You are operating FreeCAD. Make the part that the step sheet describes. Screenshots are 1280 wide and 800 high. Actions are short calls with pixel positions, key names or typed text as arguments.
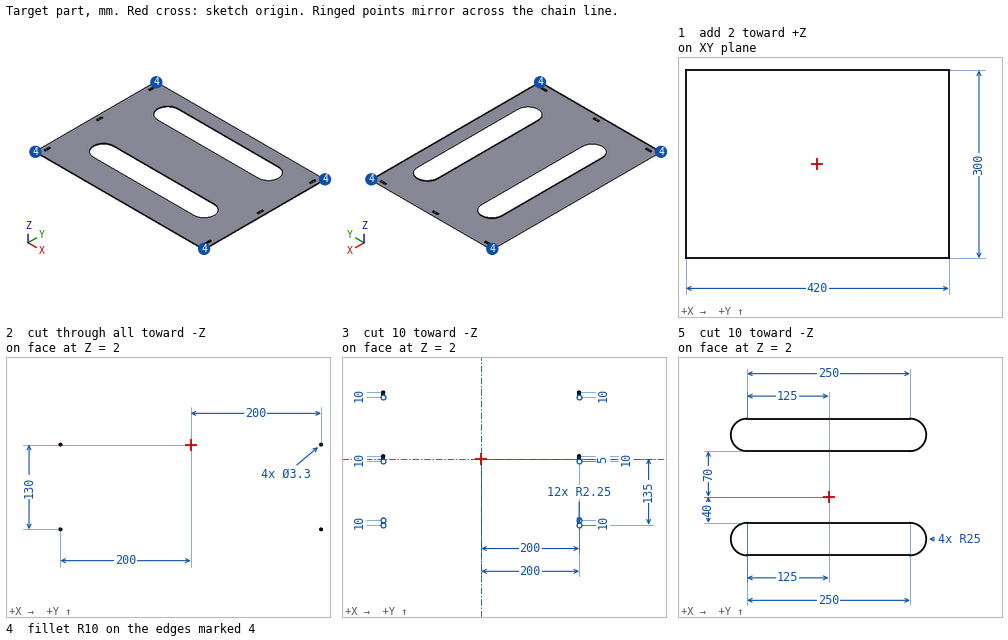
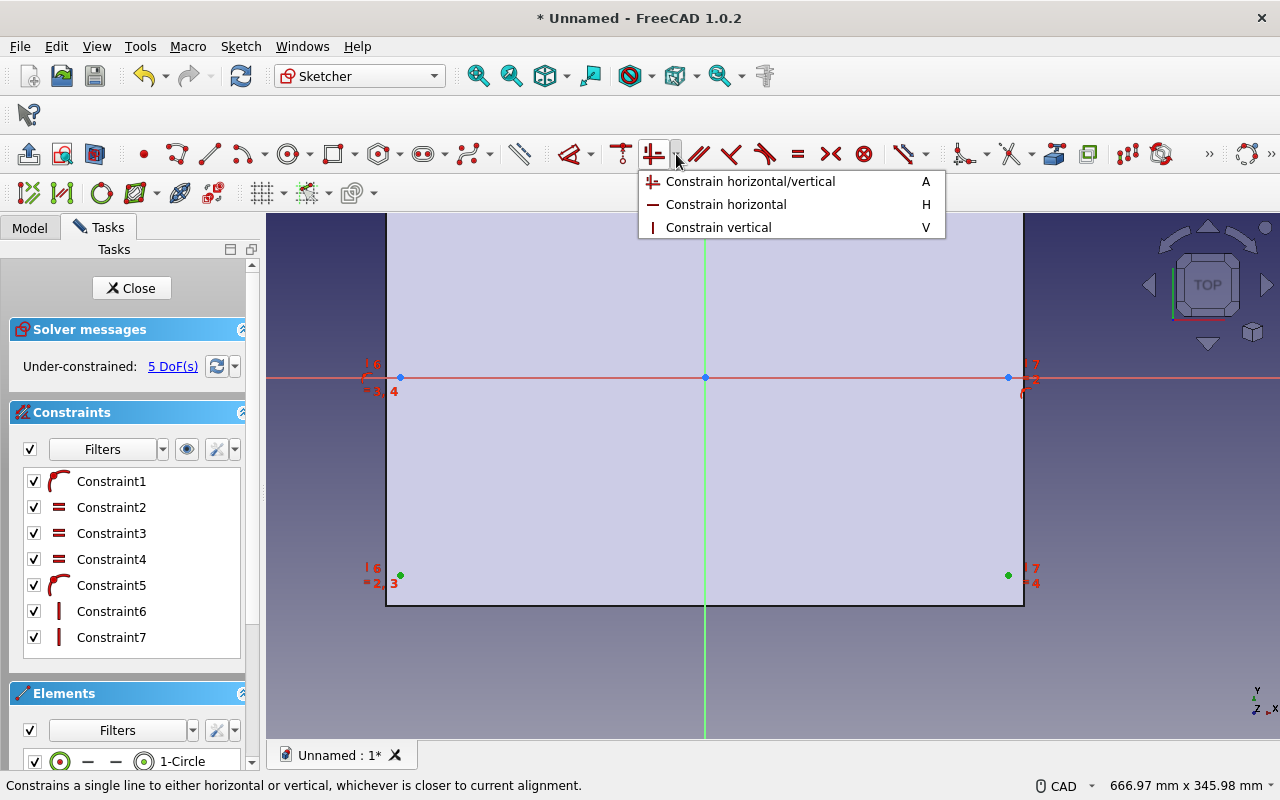
click(792, 204)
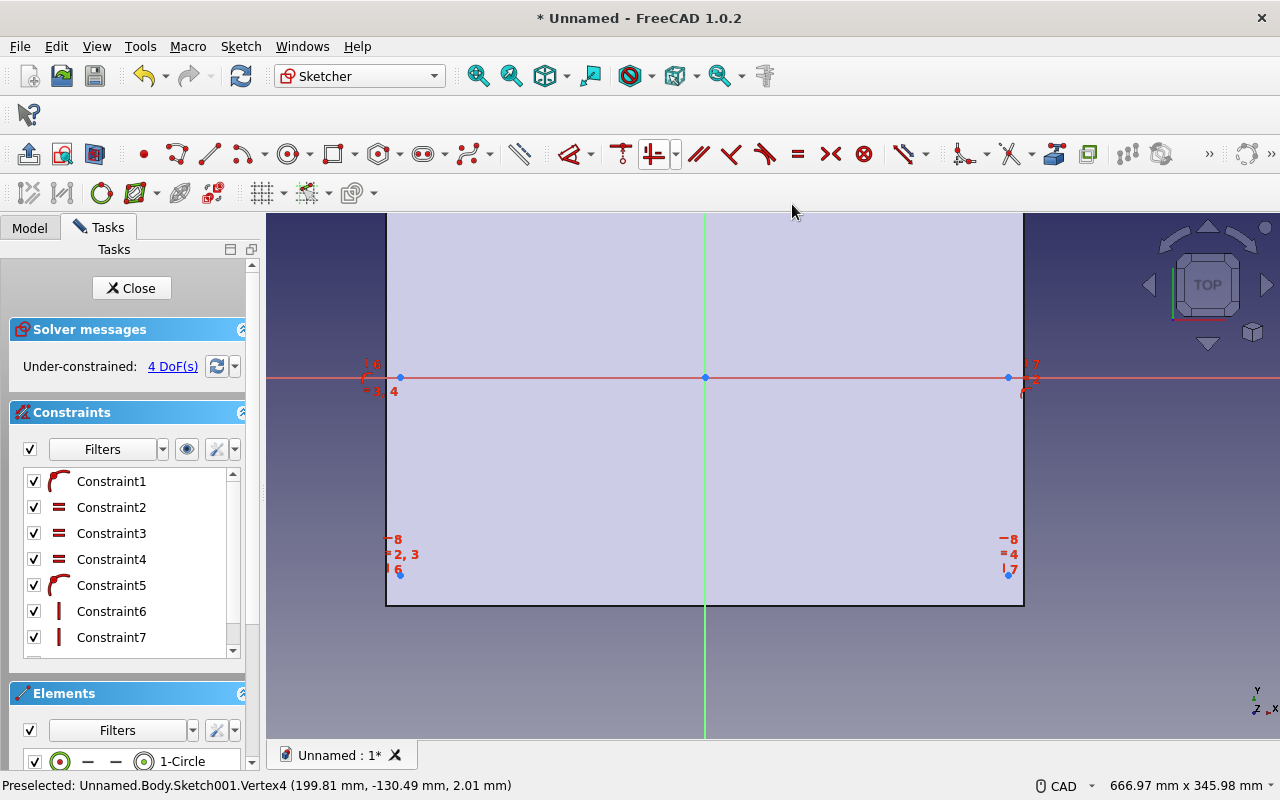
click(568, 154)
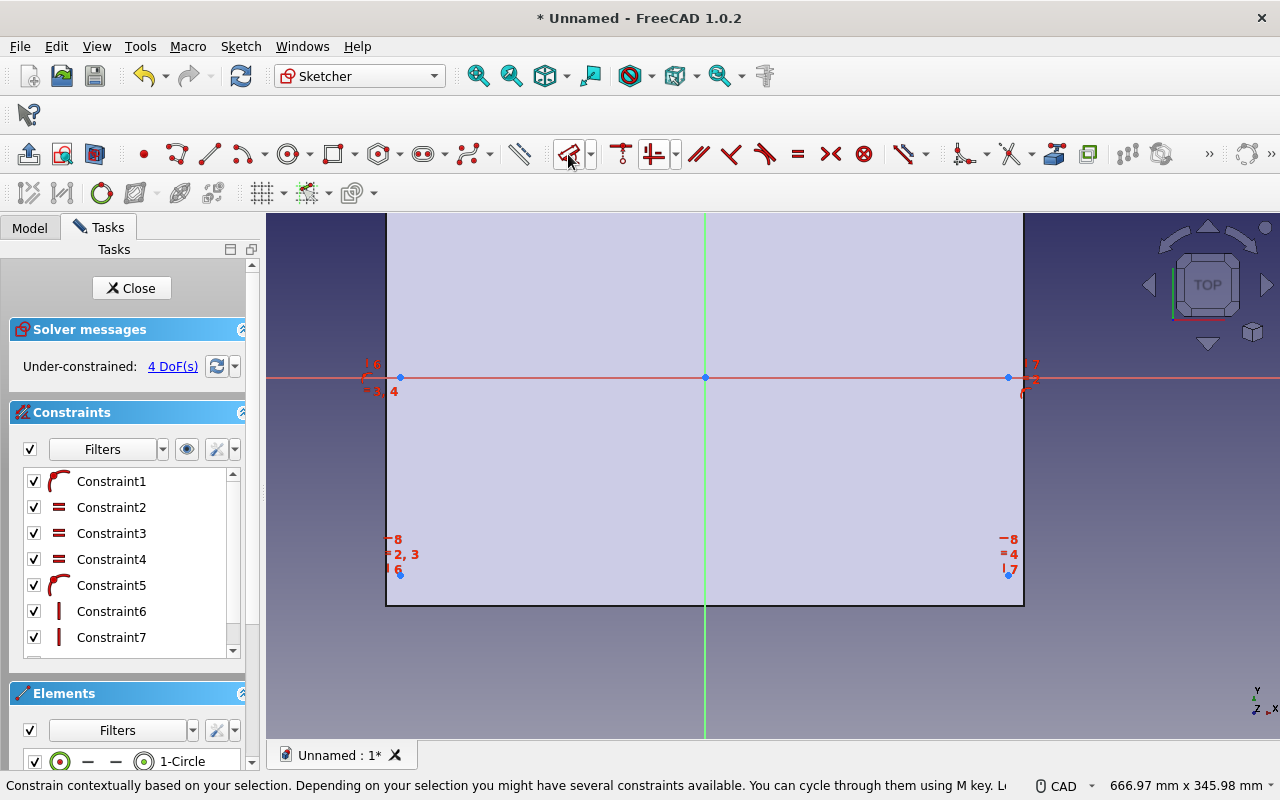
scroll(1010, 378, up, 13)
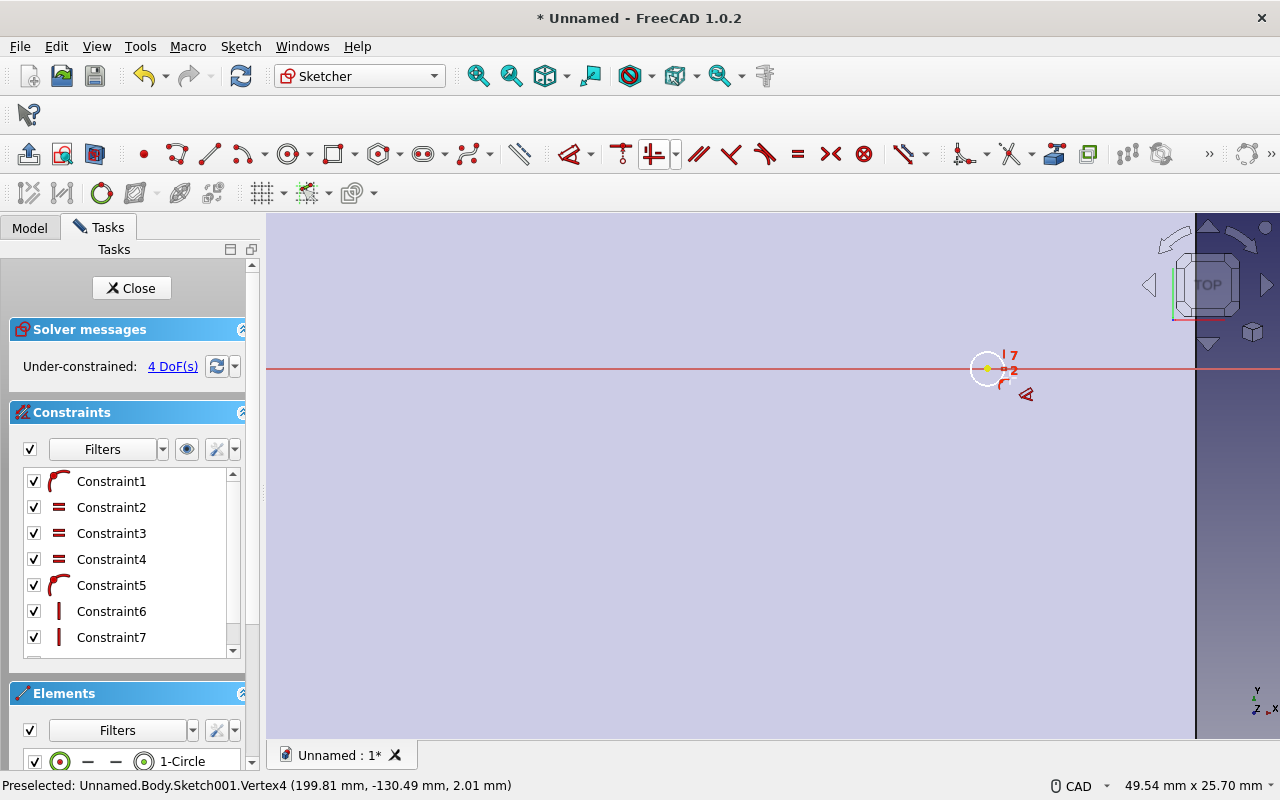
click(999, 381)
click(1021, 404)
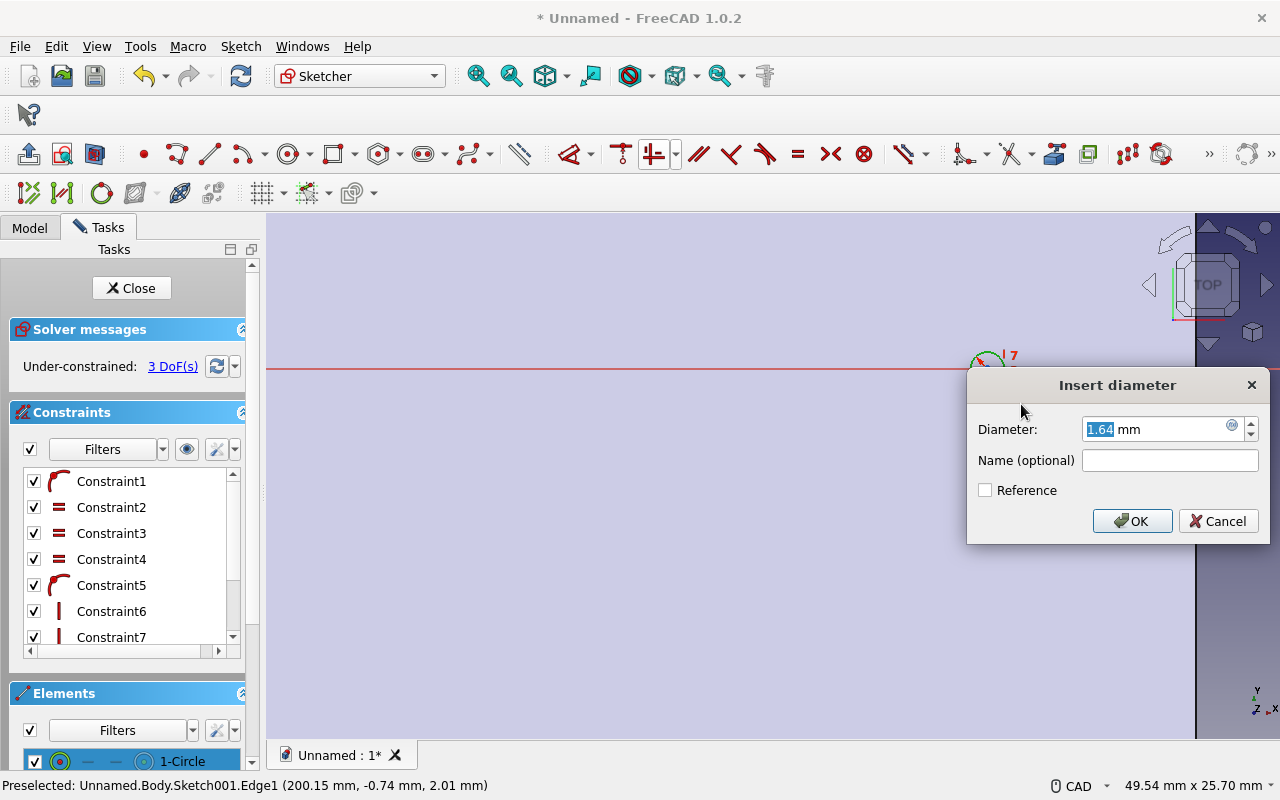
text(3.3)
key(Return)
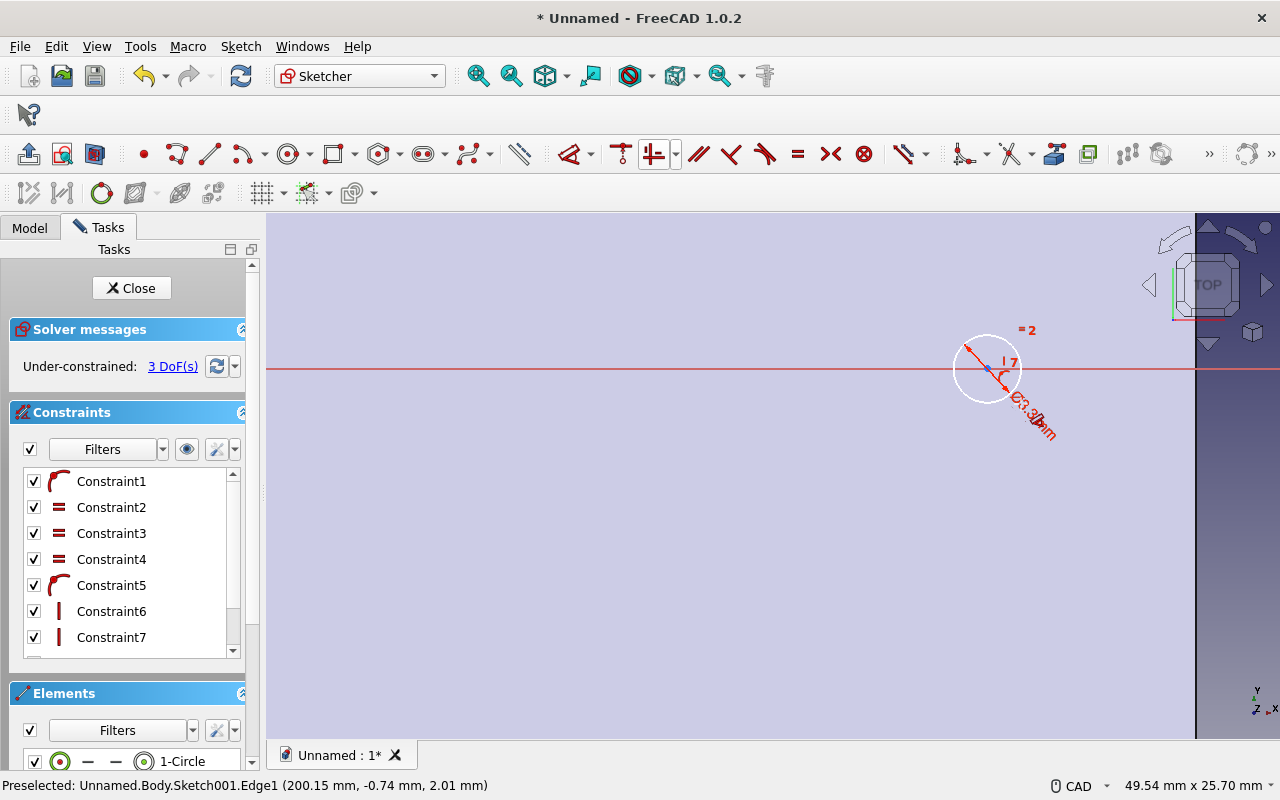
scroll(1010, 378, down, 13)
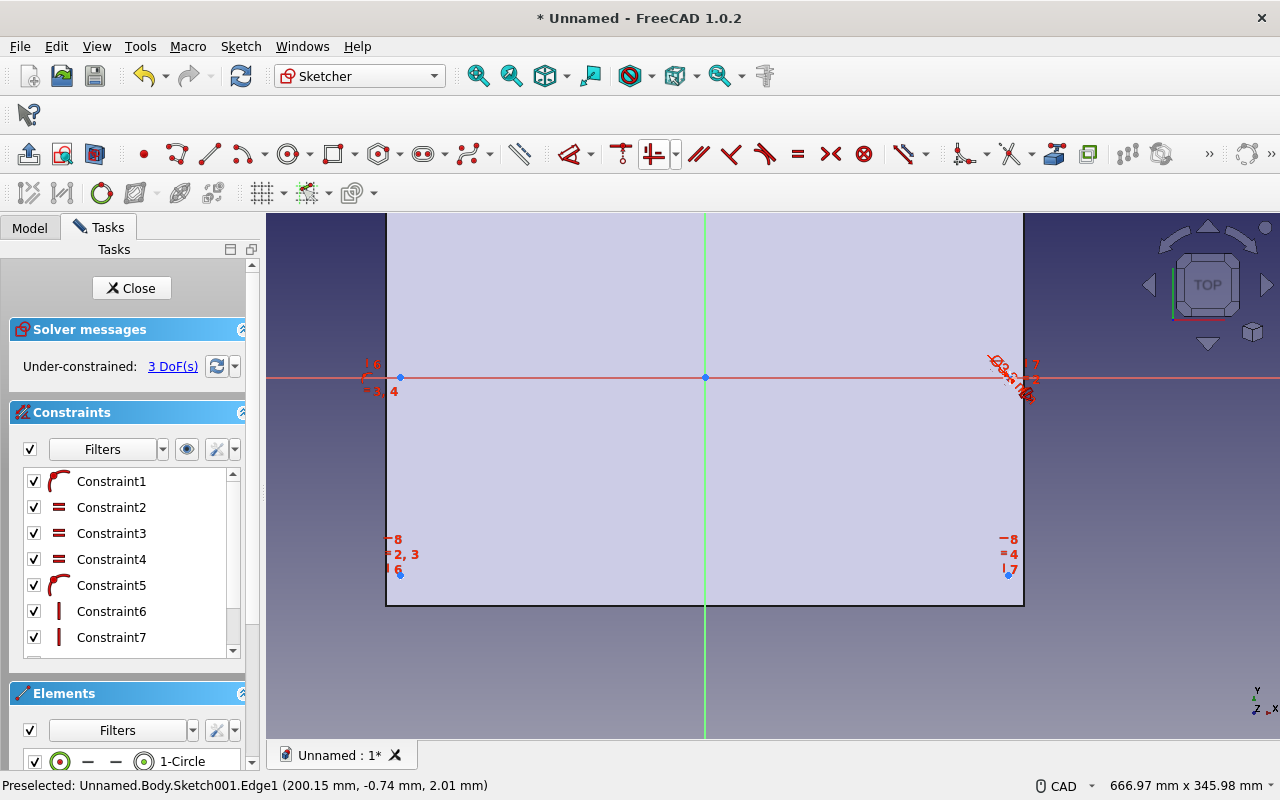
click(1009, 378)
click(857, 344)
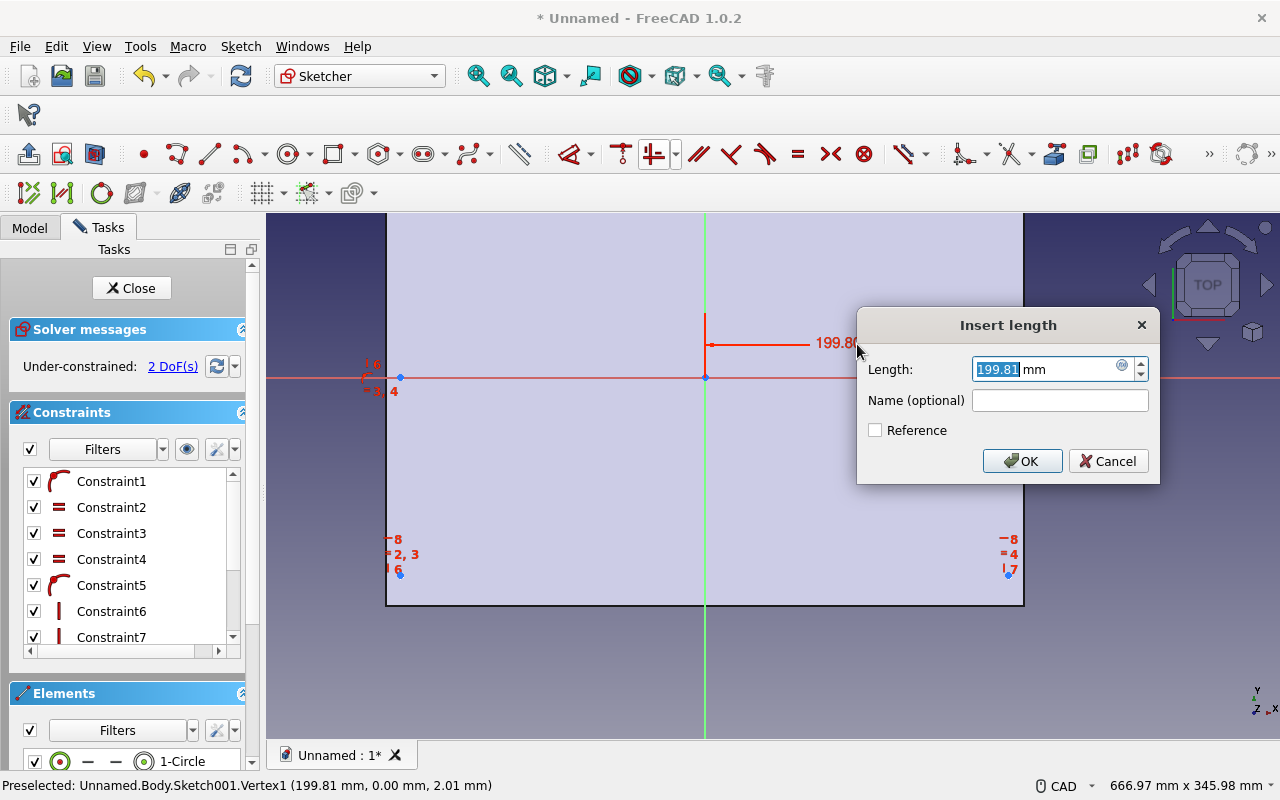
text(200)
key(Return)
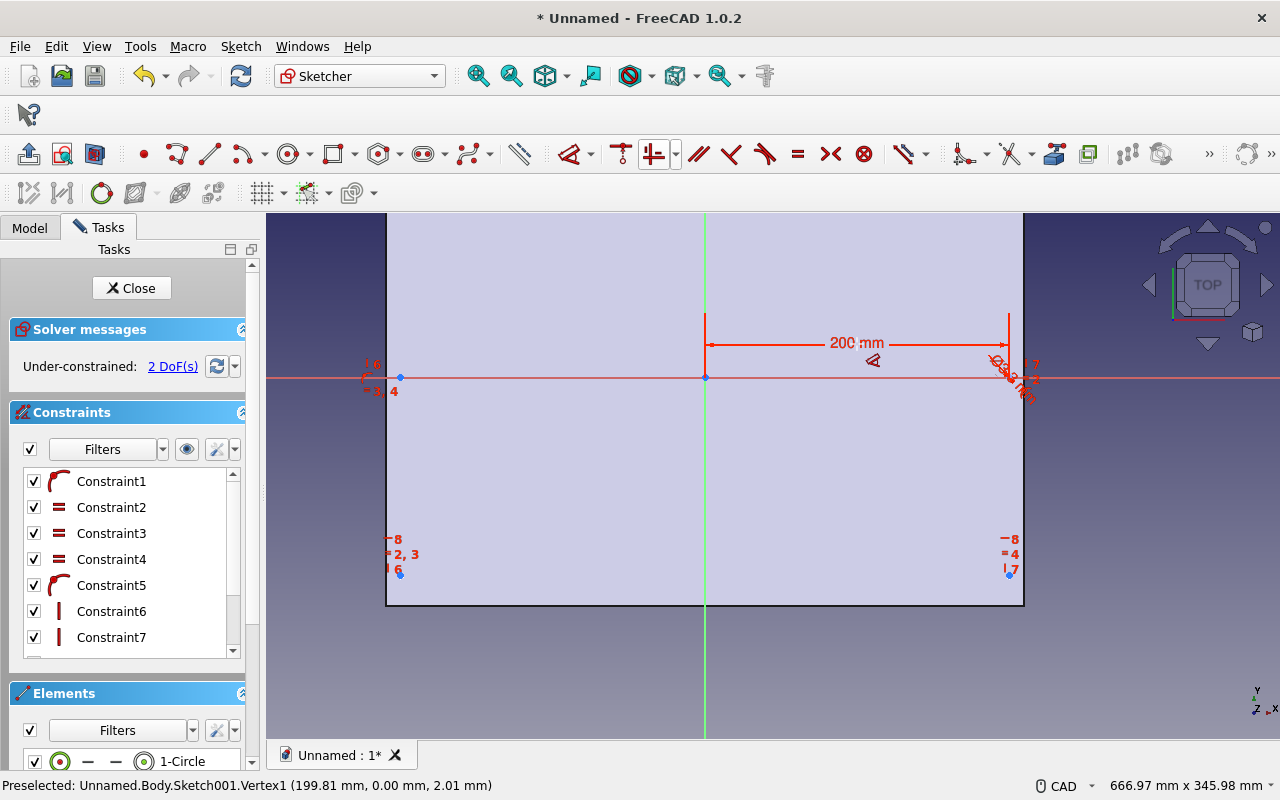
click(401, 576)
click(553, 610)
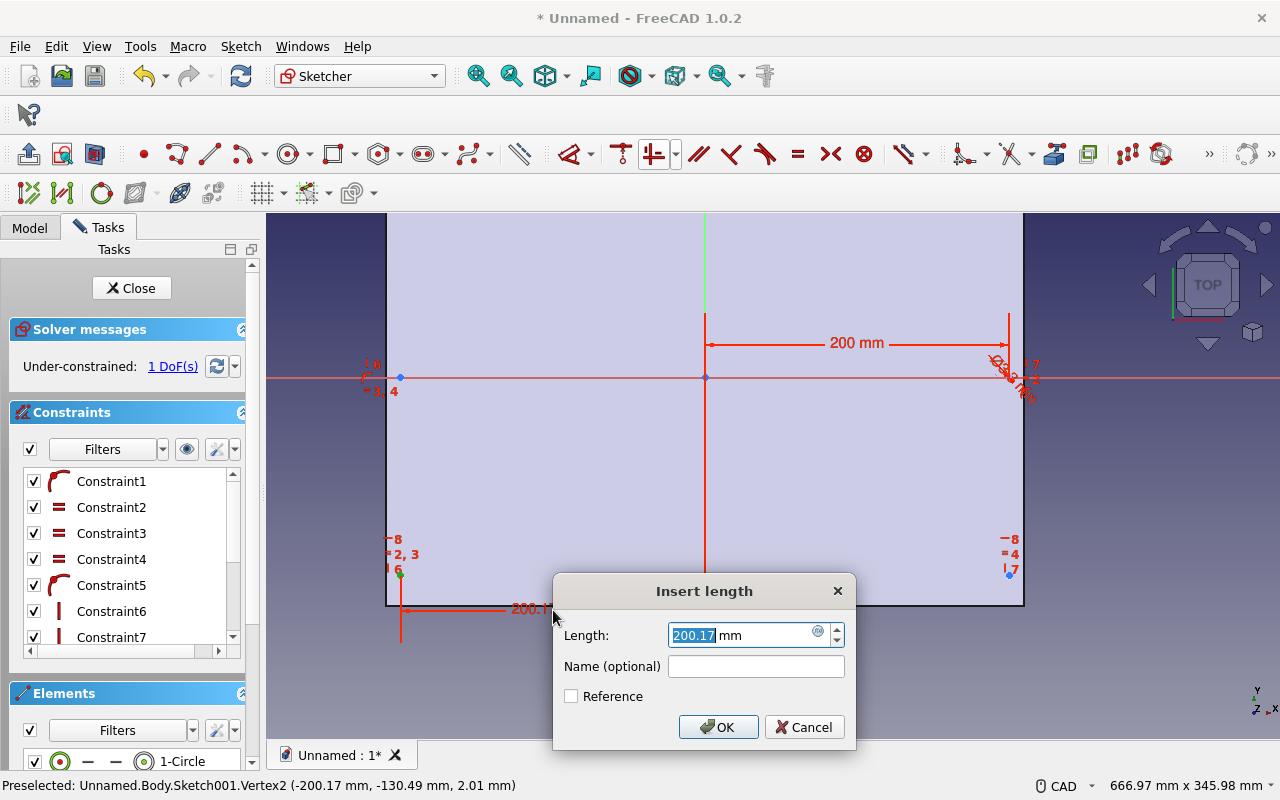
text(200)
key(Return)